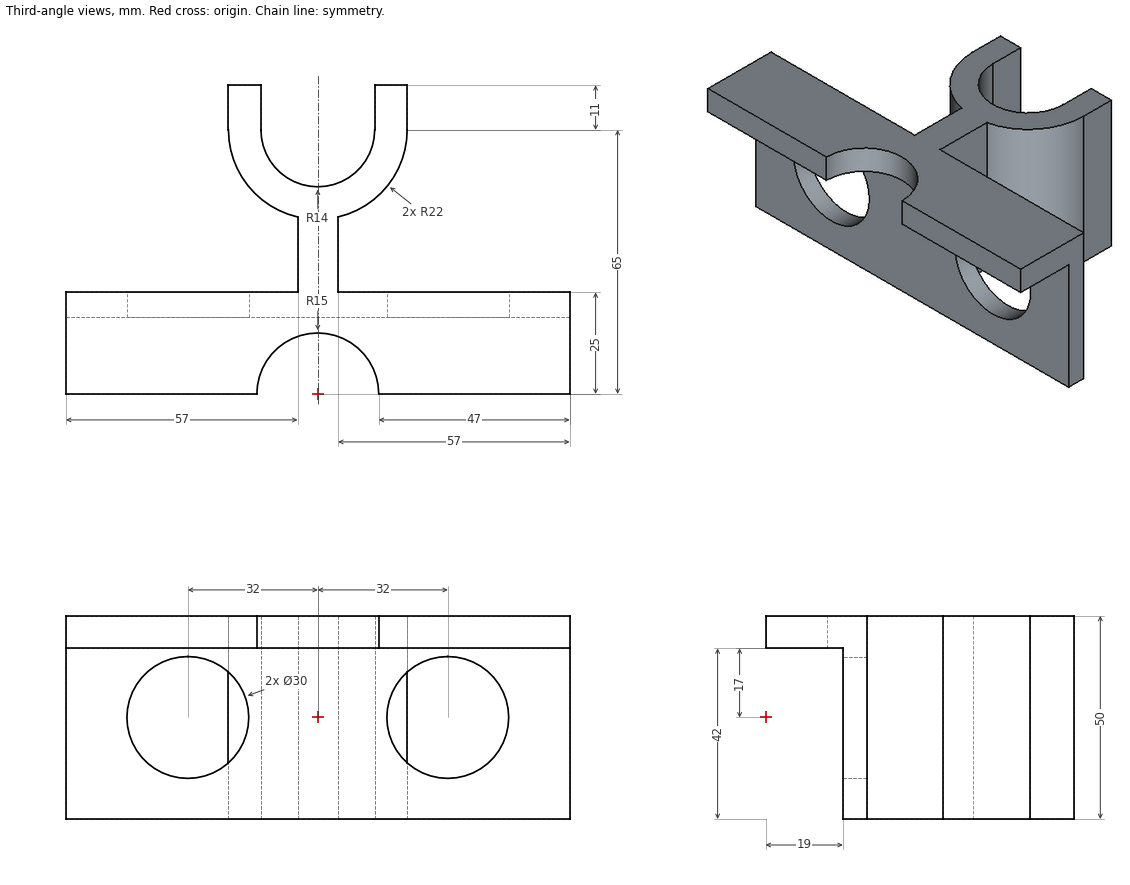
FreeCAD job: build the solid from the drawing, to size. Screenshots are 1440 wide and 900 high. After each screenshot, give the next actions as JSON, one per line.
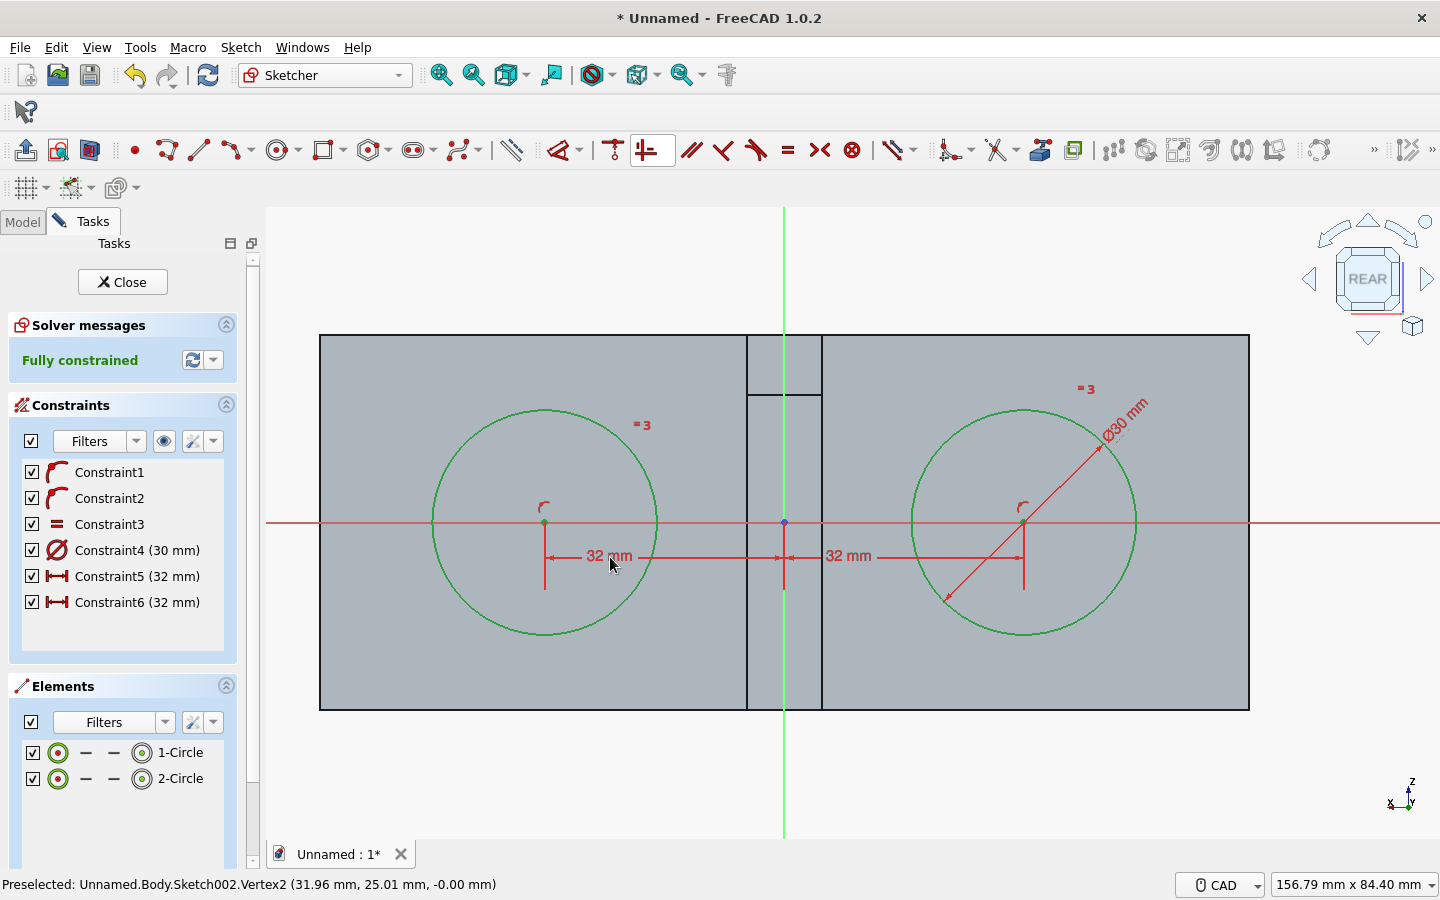
{"action": "left_click", "coordinate": [123, 282]}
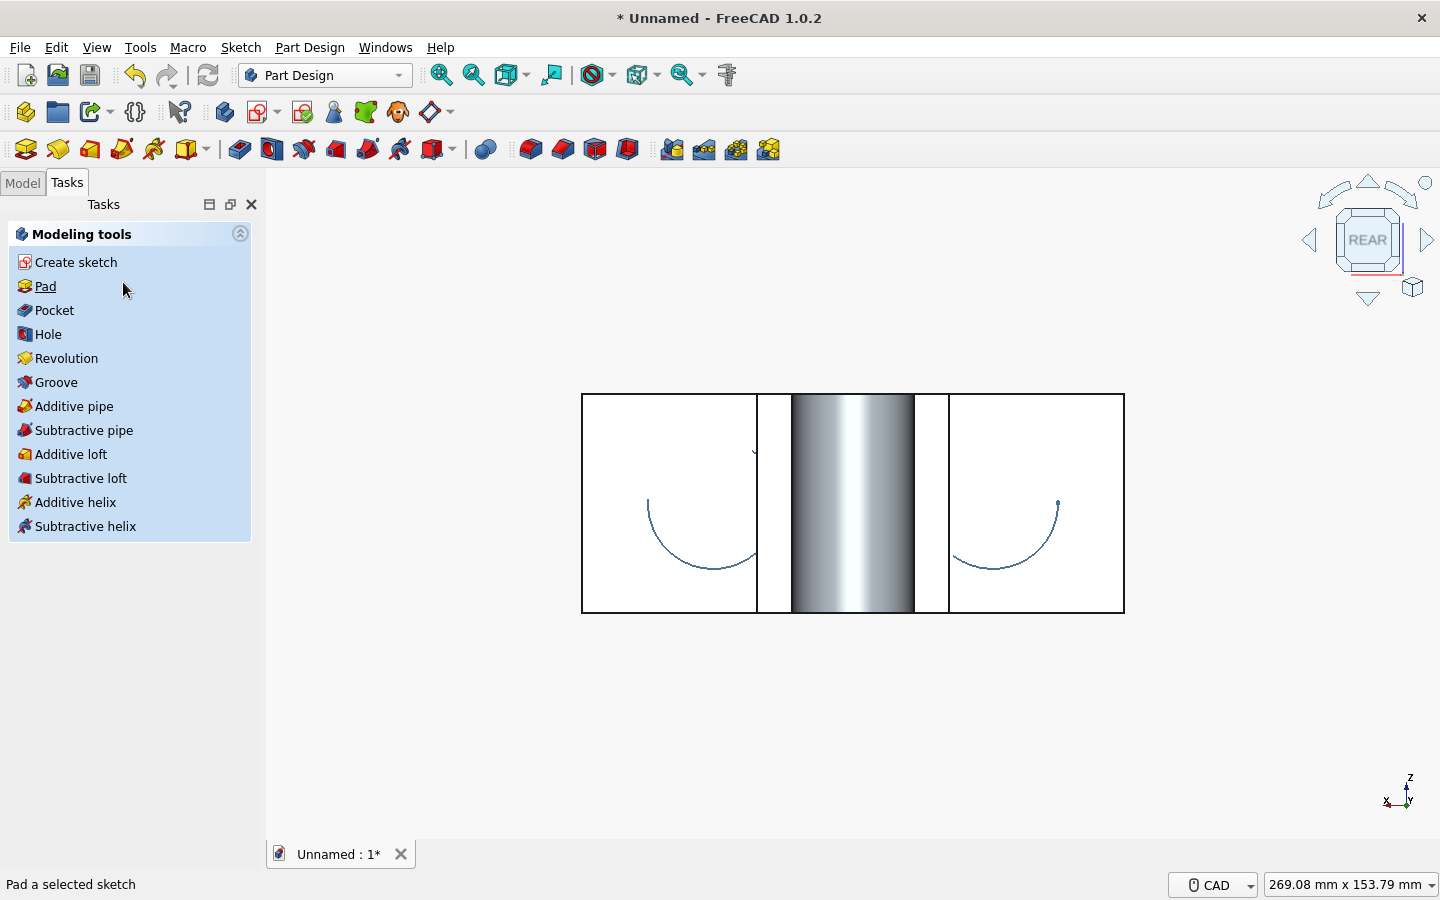
{"action": "left_click", "coordinate": [240, 150]}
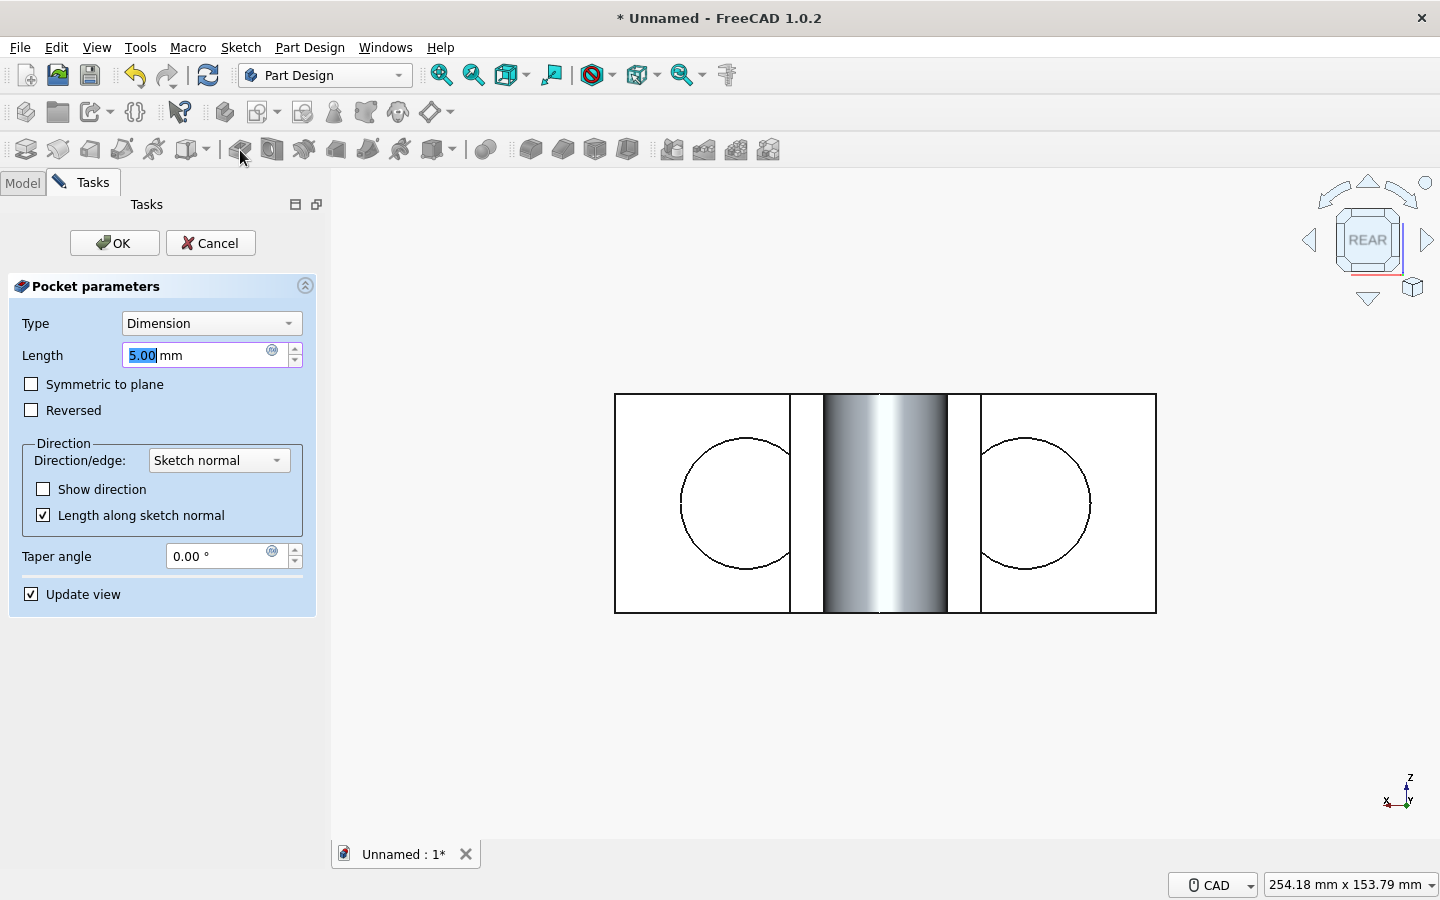
{"action": "left_click", "coordinate": [212, 324]}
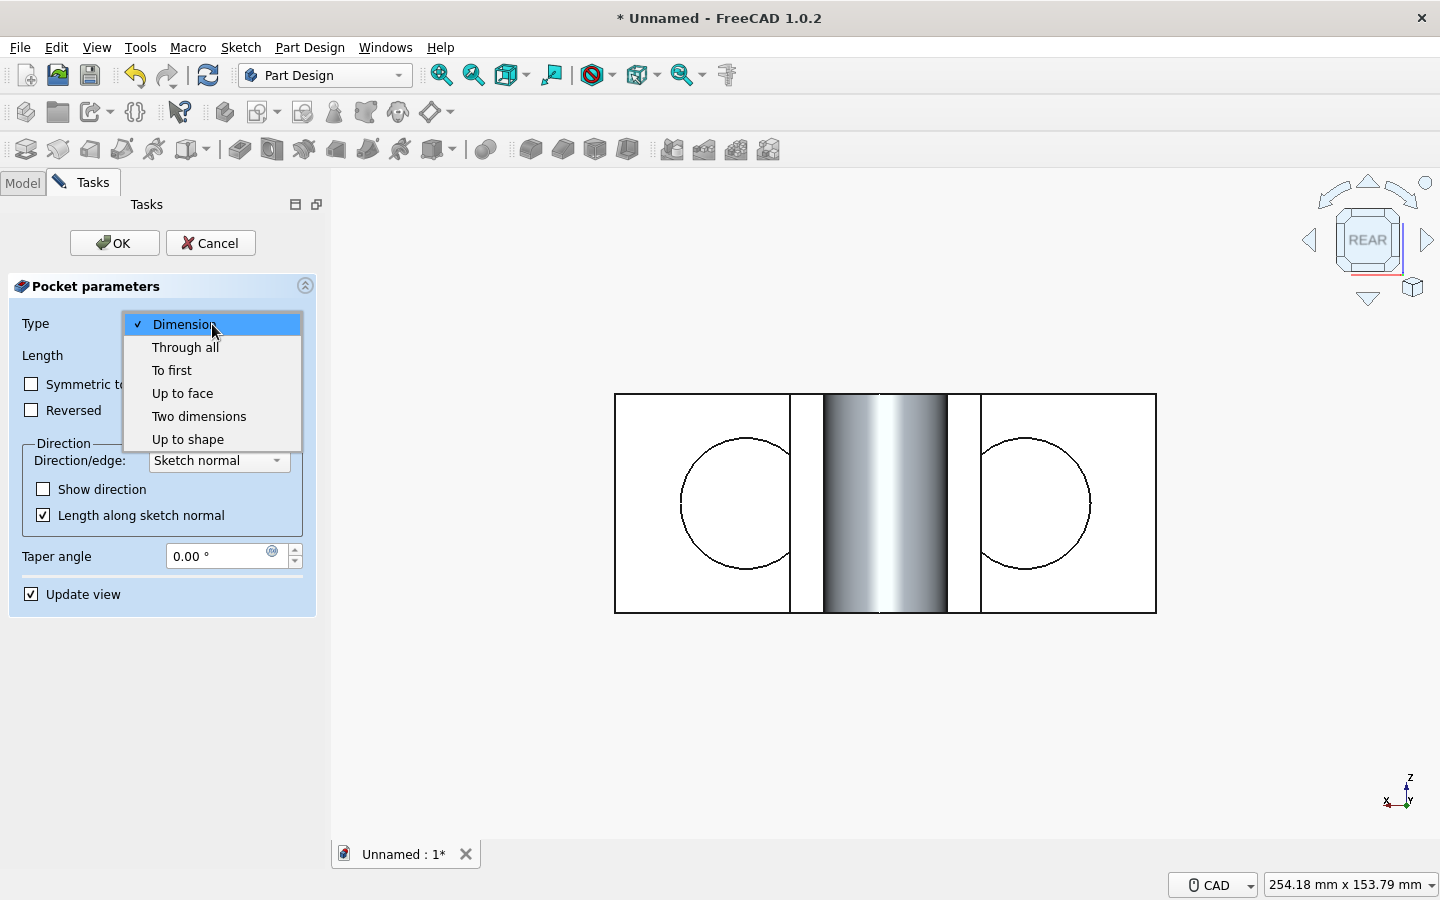
{"action": "left_click", "coordinate": [212, 348]}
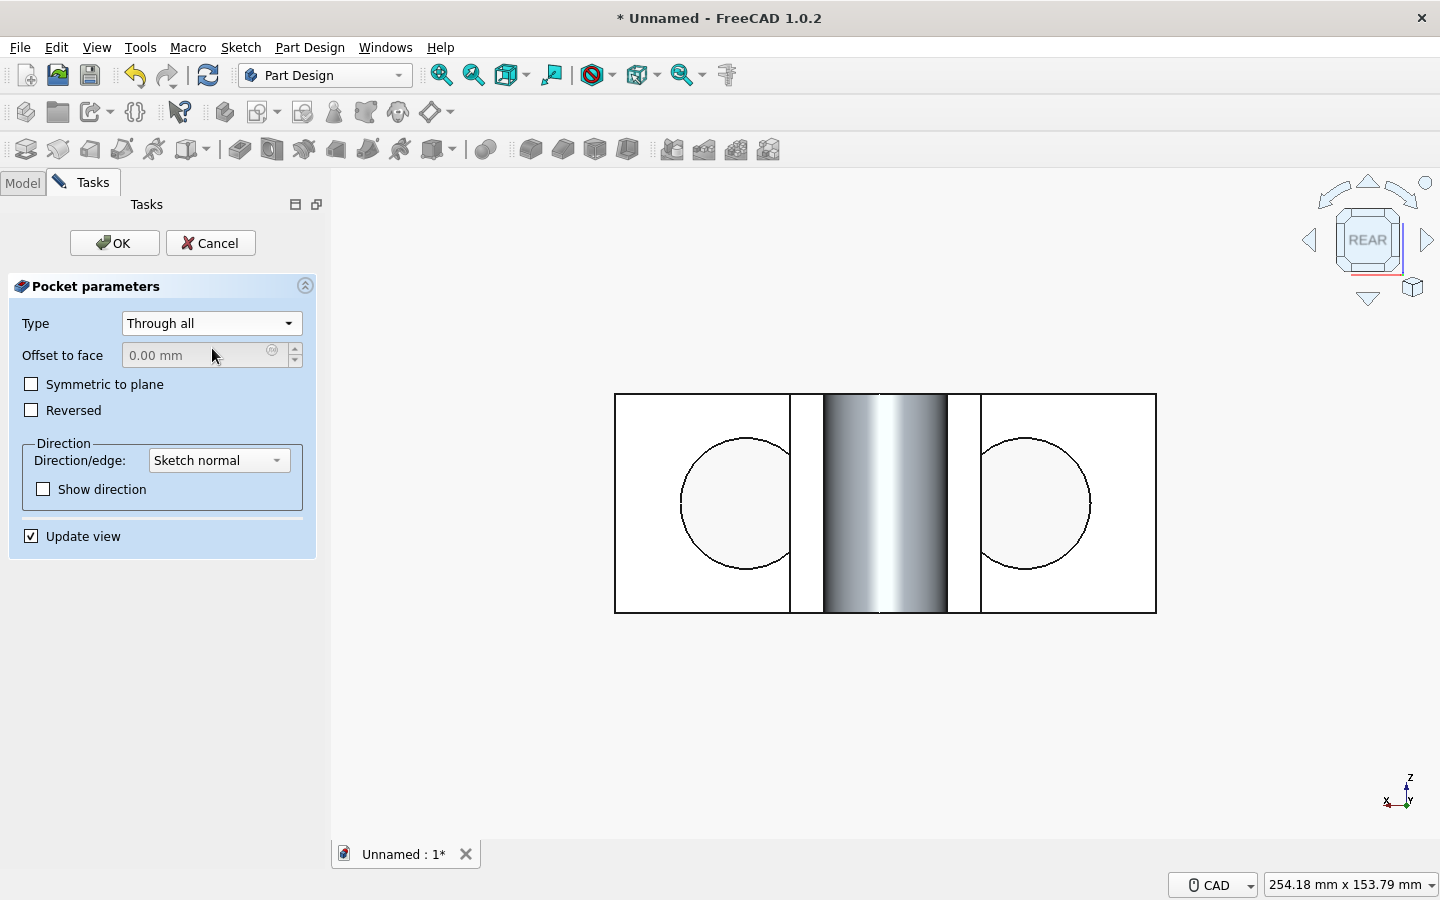
{"action": "left_click", "coordinate": [115, 243]}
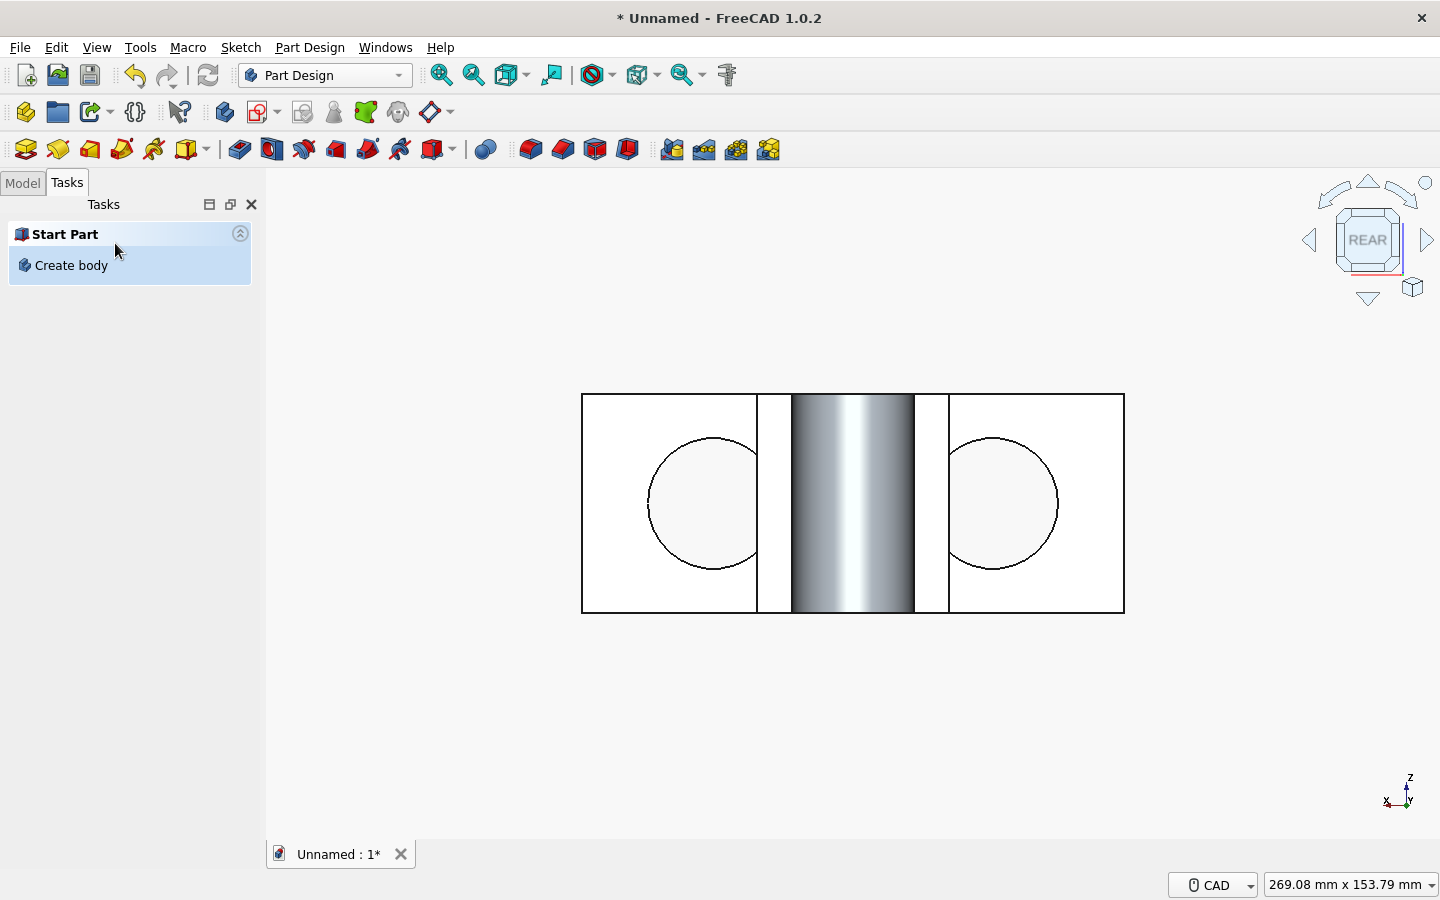
{"action": "key", "text": "0"}